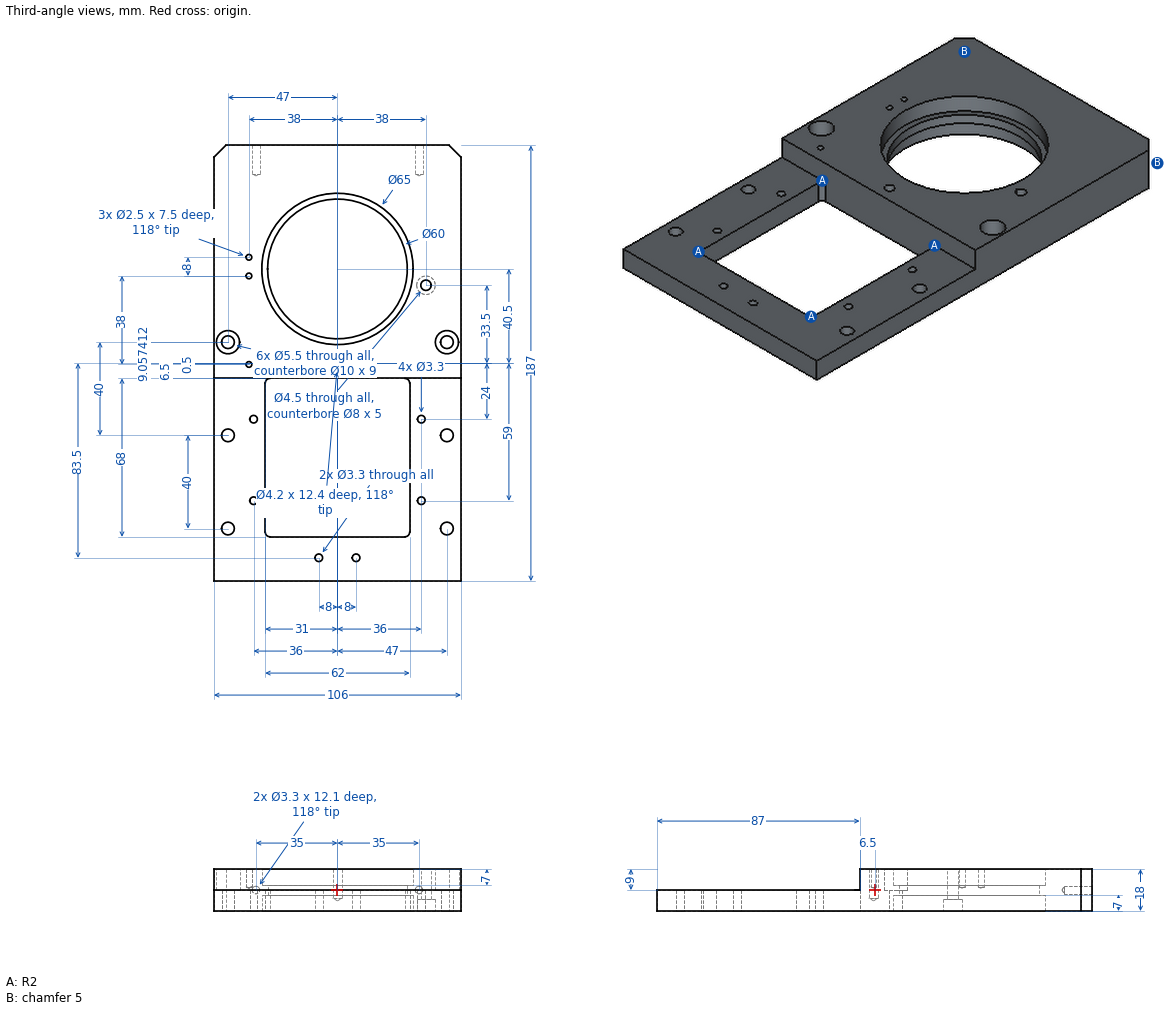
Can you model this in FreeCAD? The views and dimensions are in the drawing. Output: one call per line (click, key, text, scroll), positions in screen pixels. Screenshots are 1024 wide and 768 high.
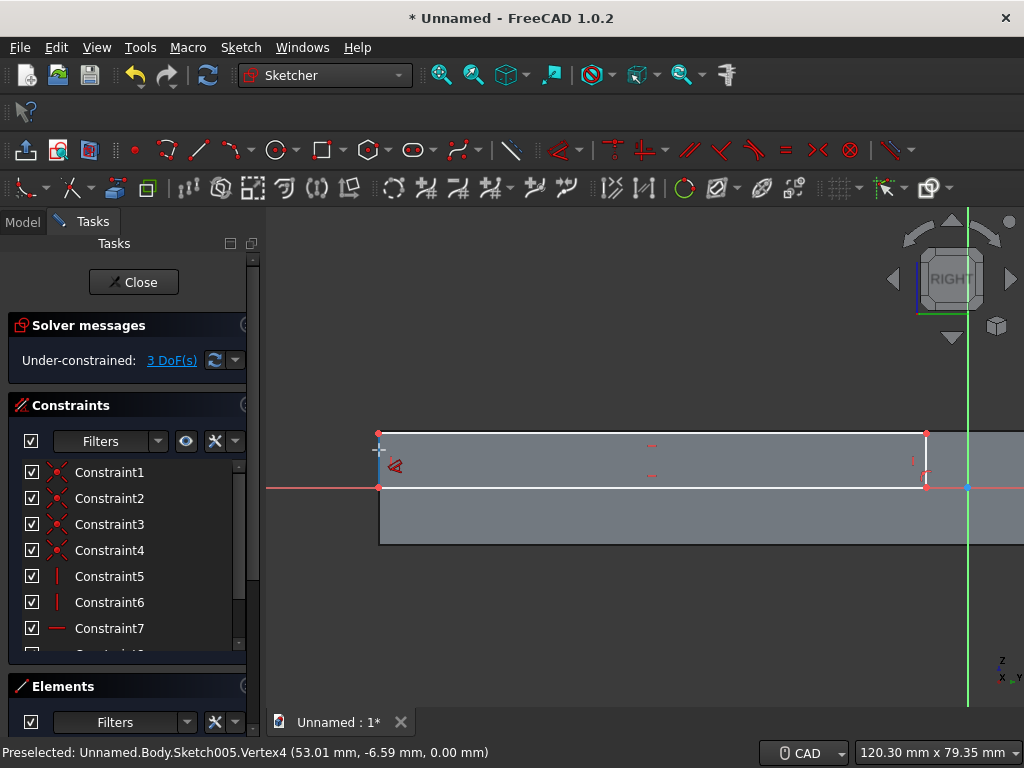
click(379, 450)
click(345, 461)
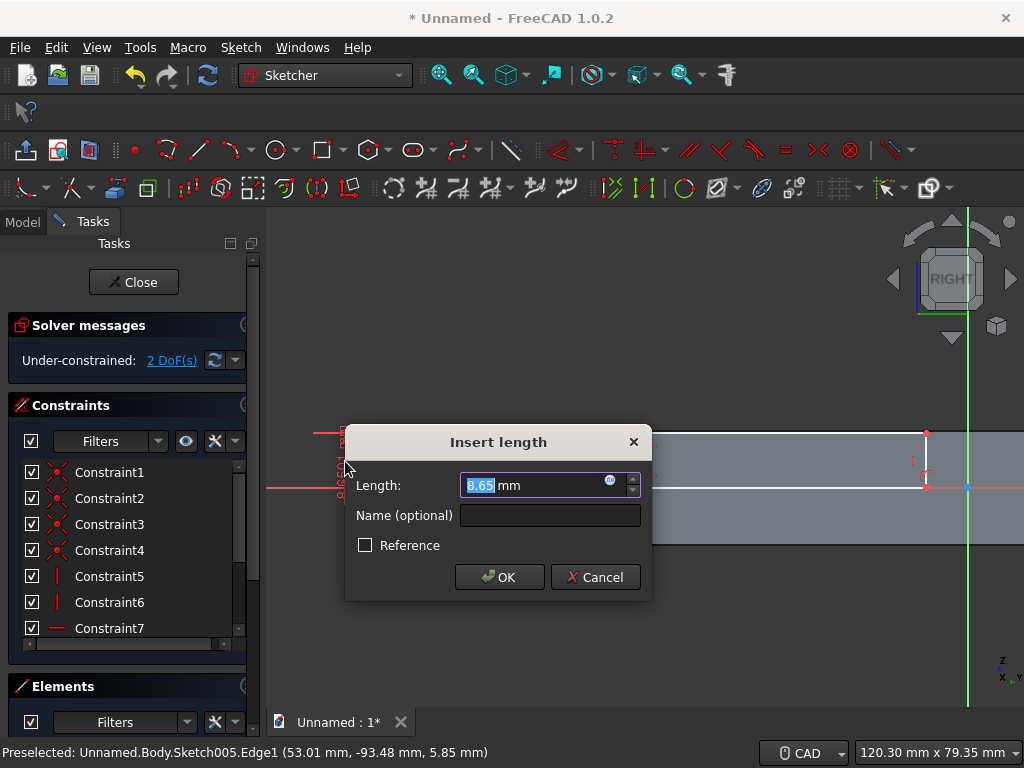
text(9)
key(Return)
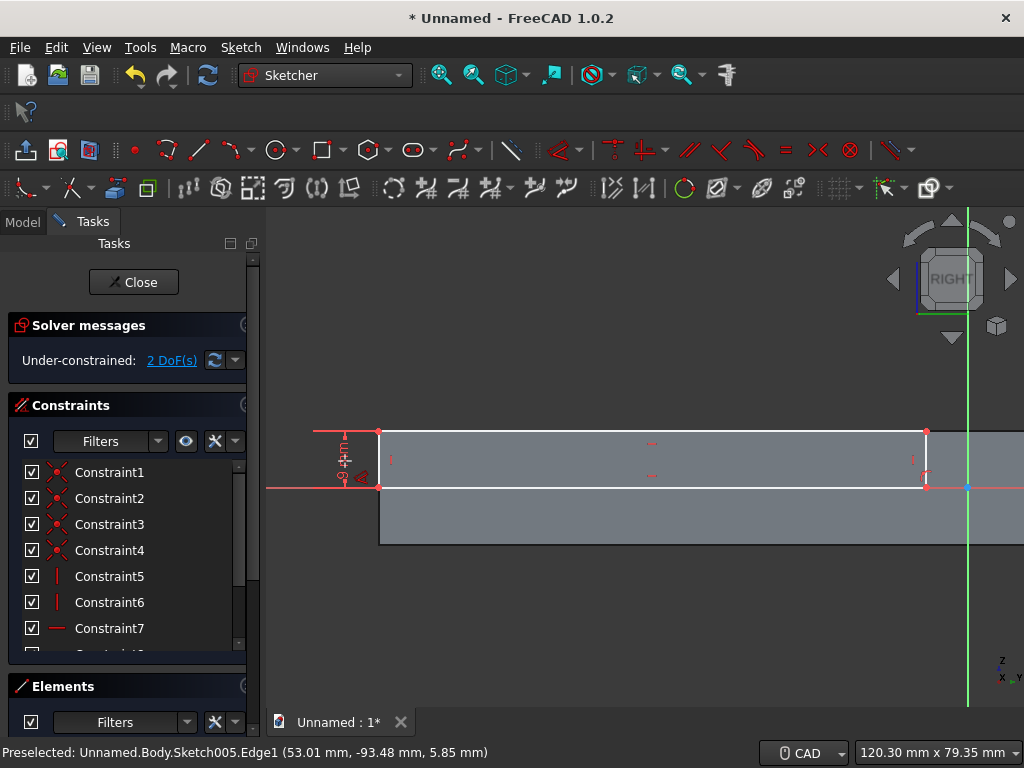
click(543, 488)
click(619, 522)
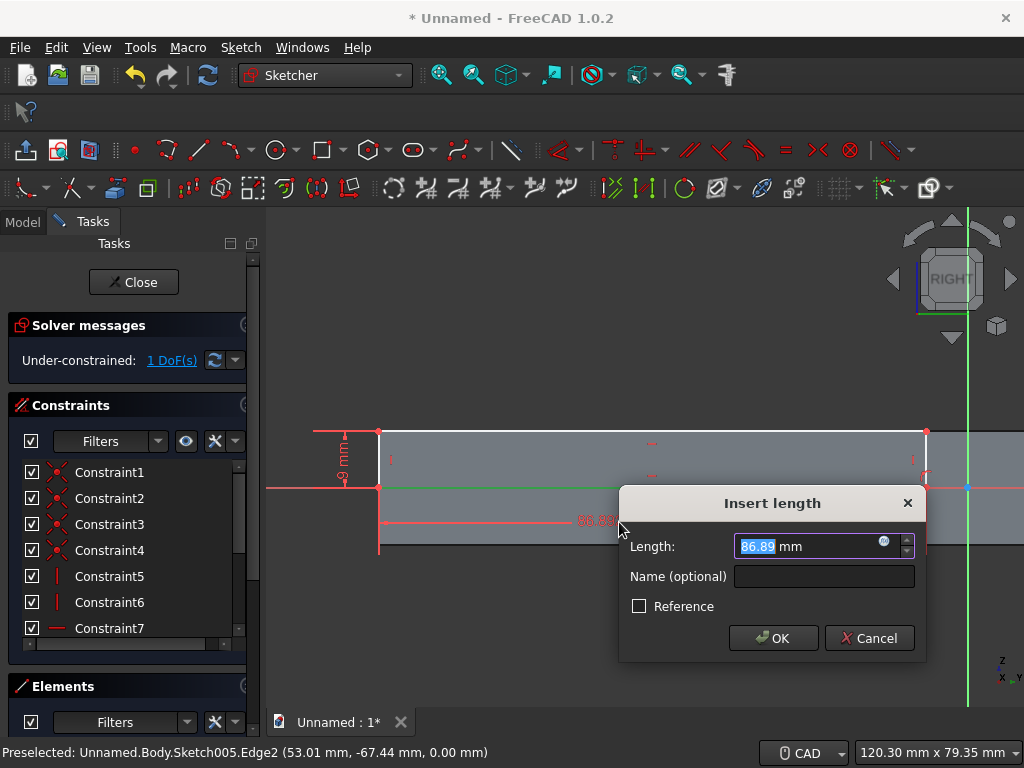
text(87)
key(Return)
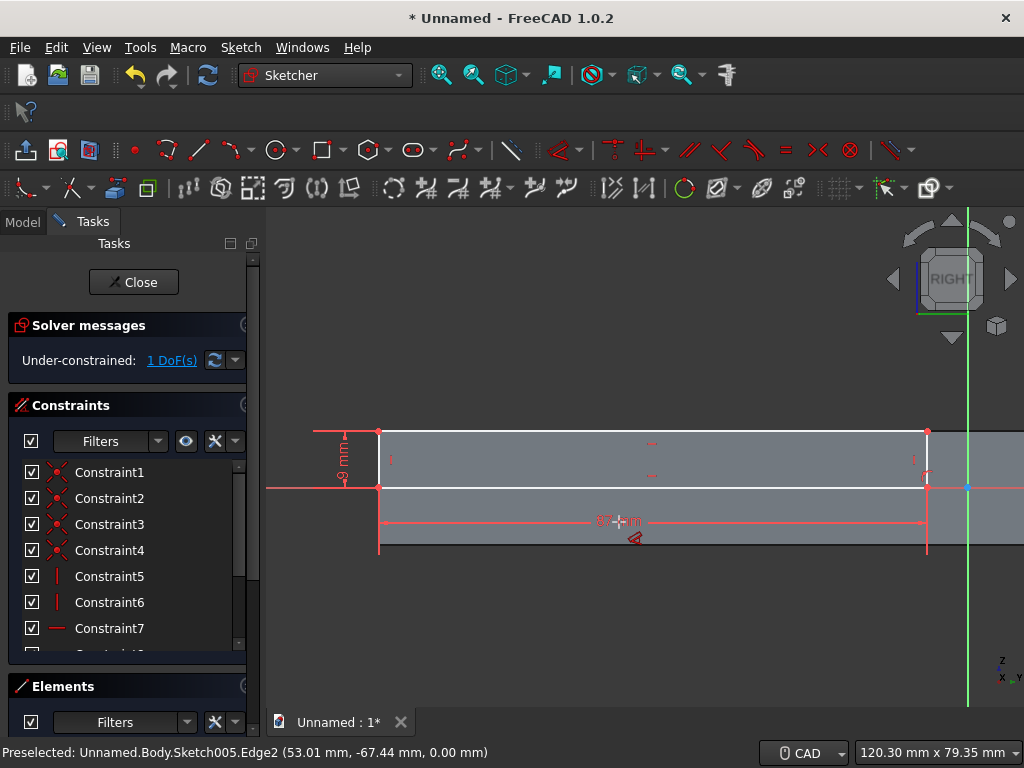
scroll(380, 452, down, 2)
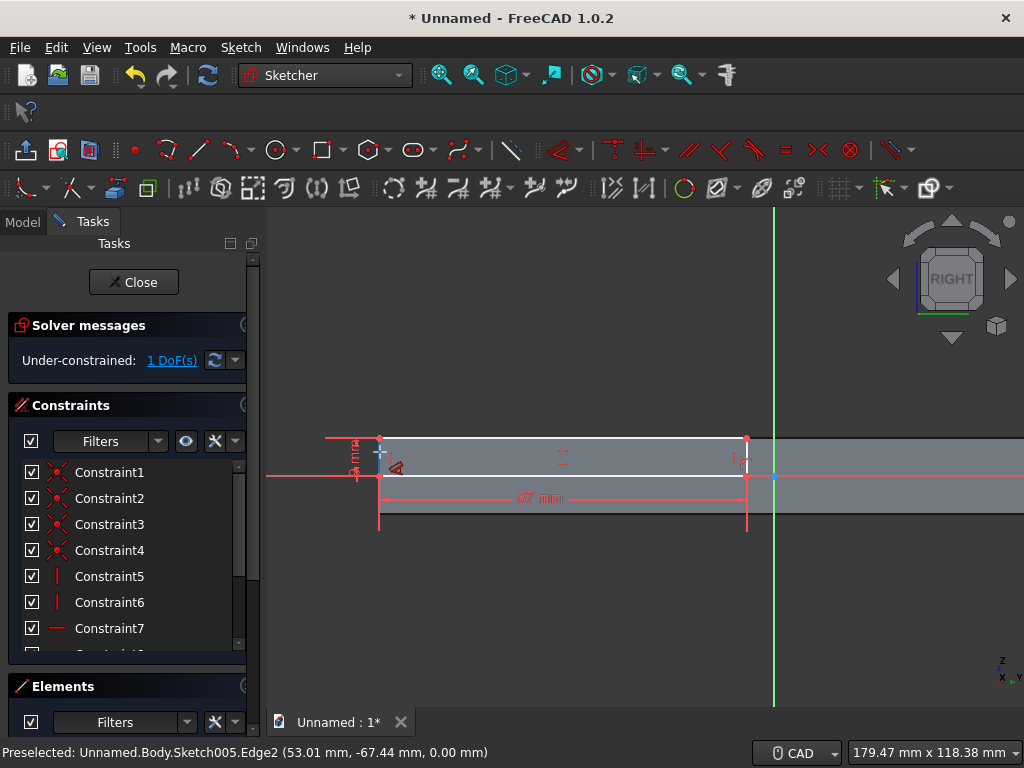
scroll(747, 476, up, 2)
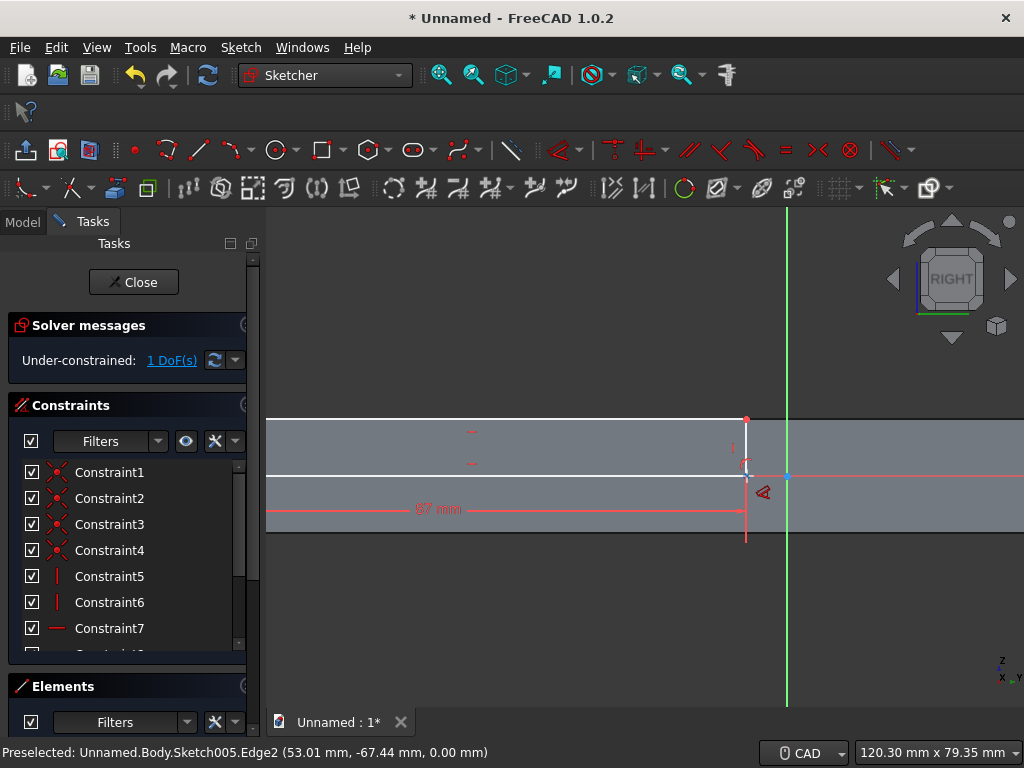
click(746, 476)
click(767, 510)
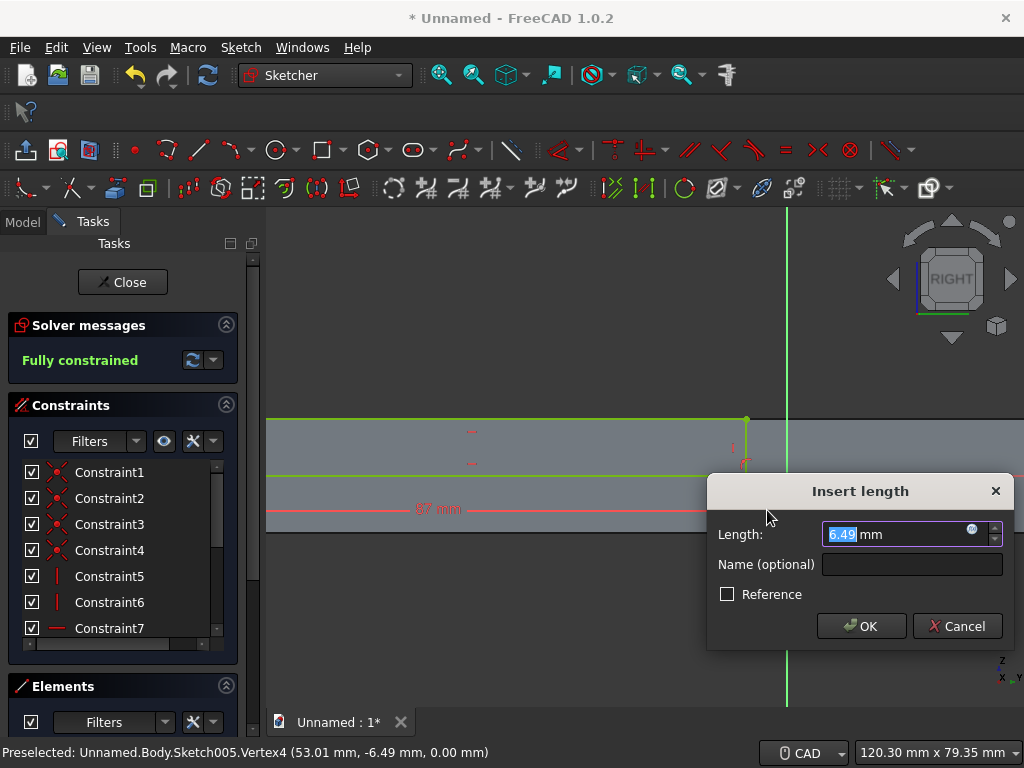
text(6.5)
key(Return)
key(Escape)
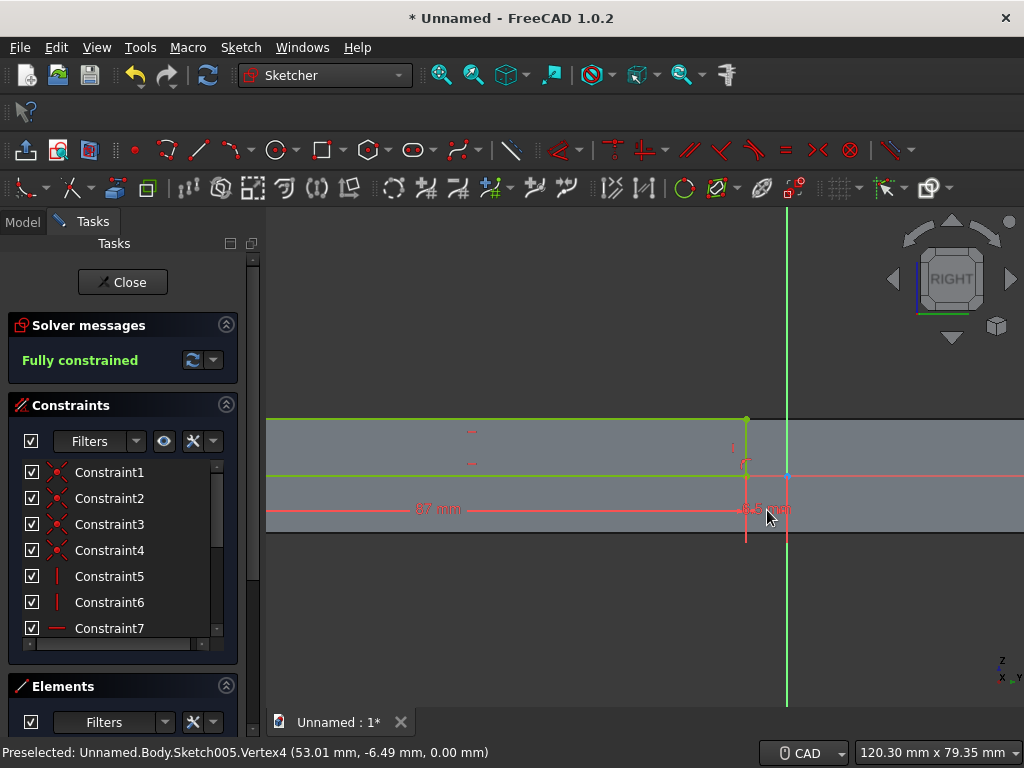
click(123, 282)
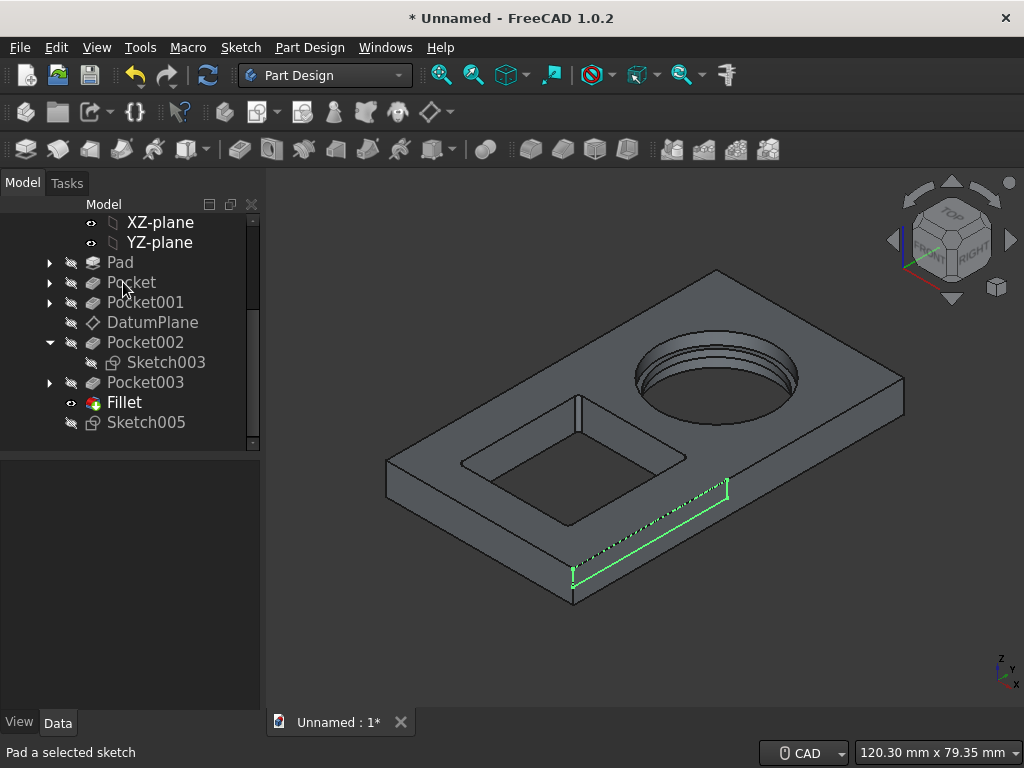
click(240, 150)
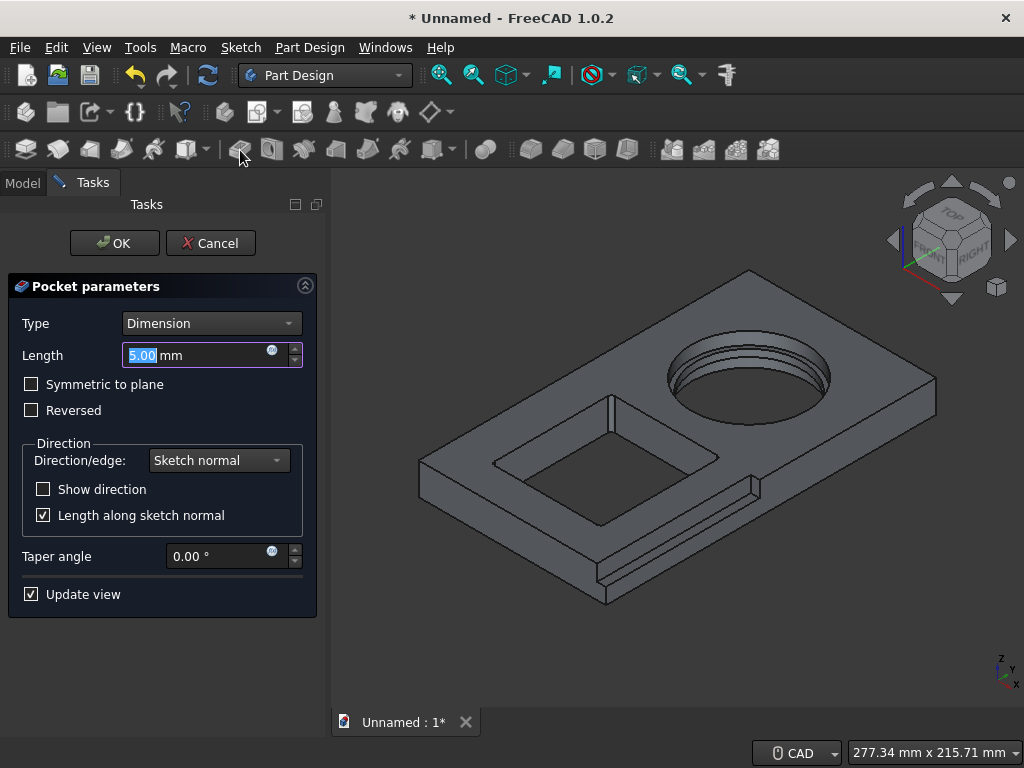
click(212, 324)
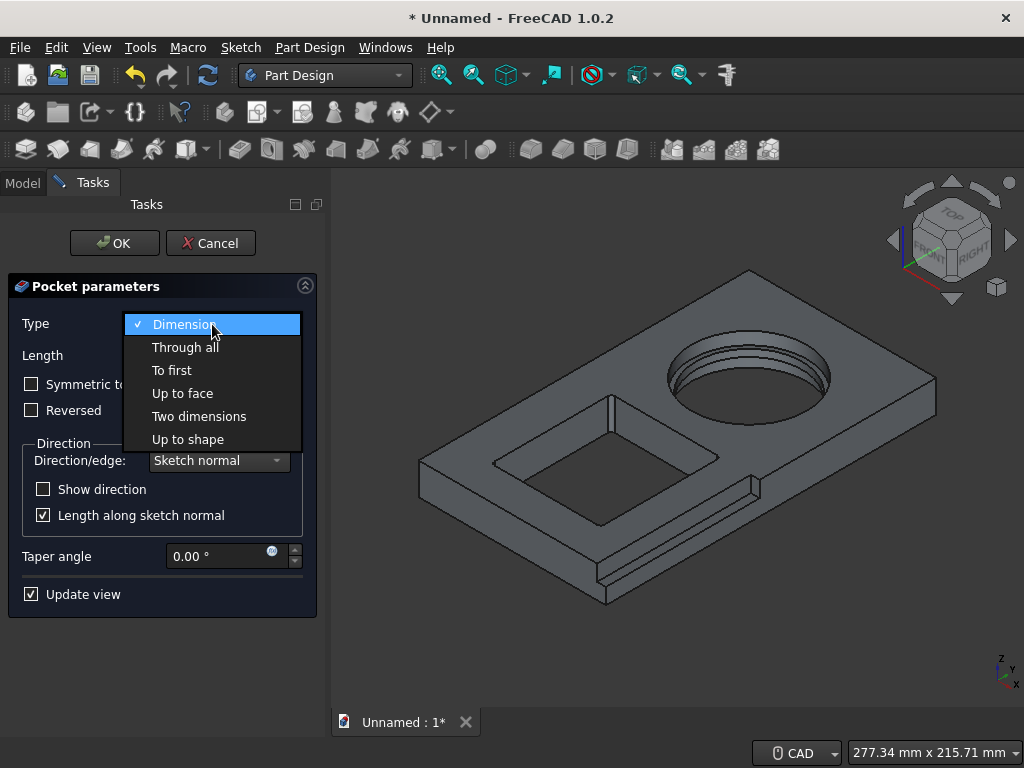
click(212, 348)